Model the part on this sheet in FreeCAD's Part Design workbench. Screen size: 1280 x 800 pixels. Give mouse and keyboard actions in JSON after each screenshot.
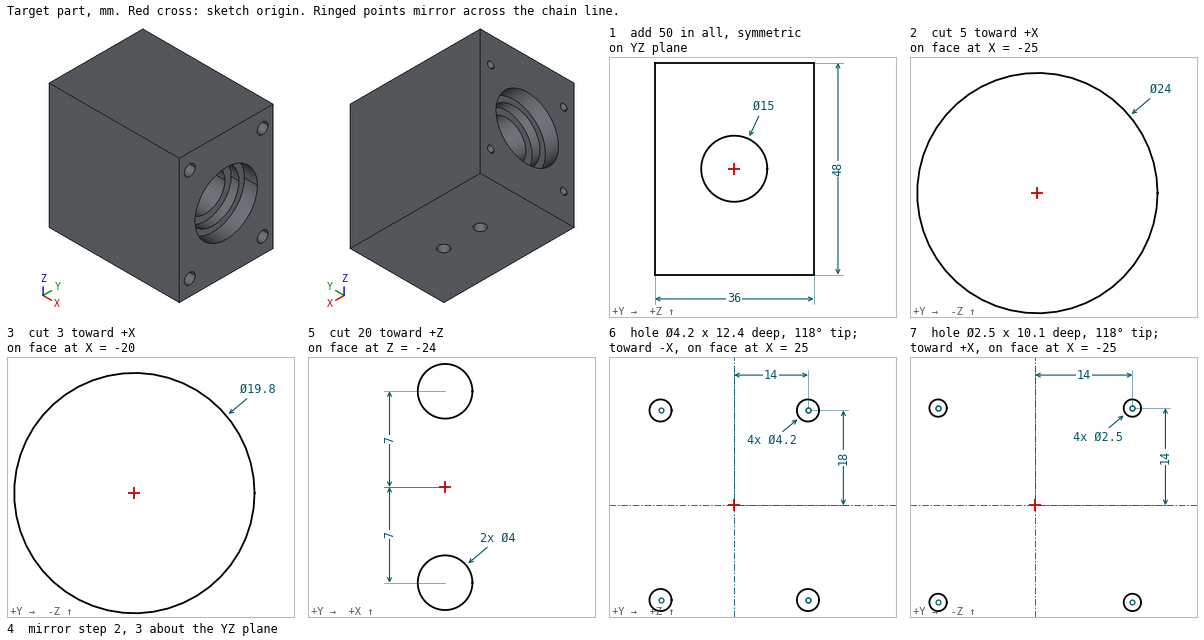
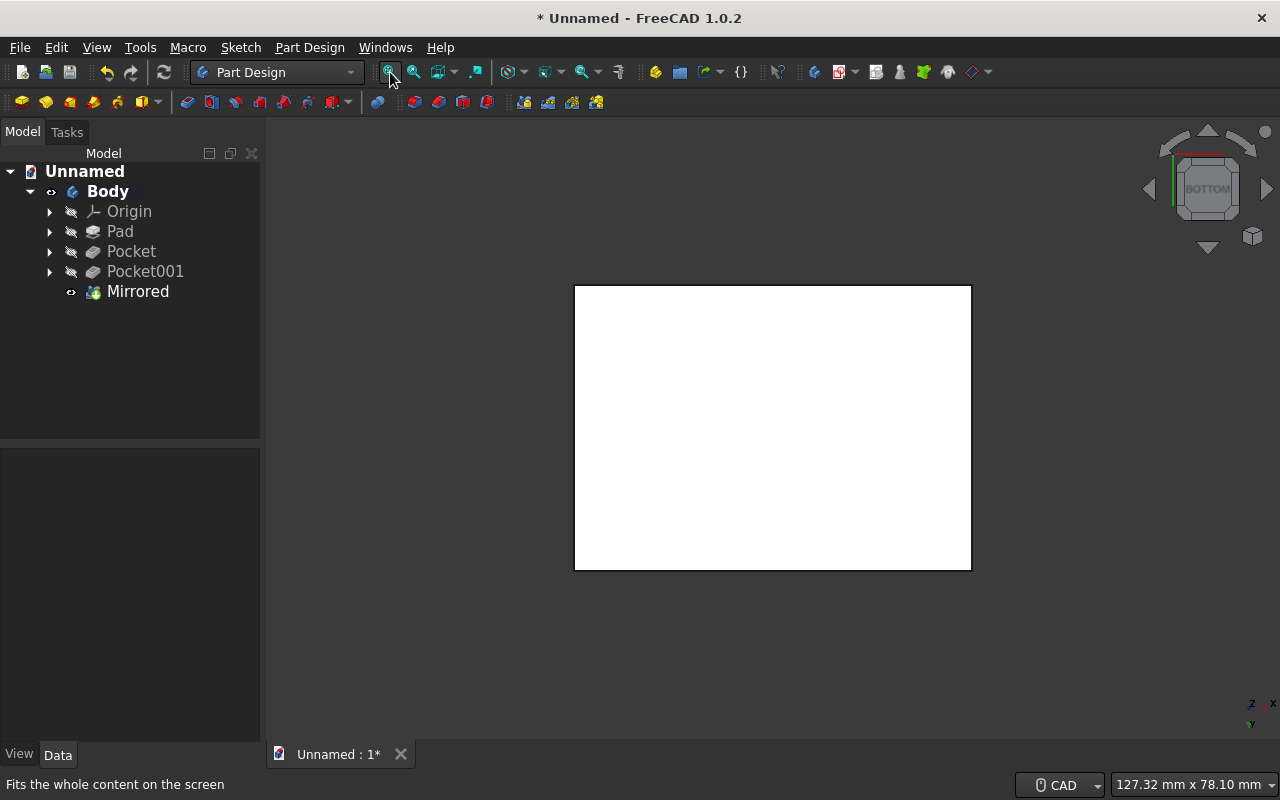
{"action": "left_click", "coordinate": [773, 427]}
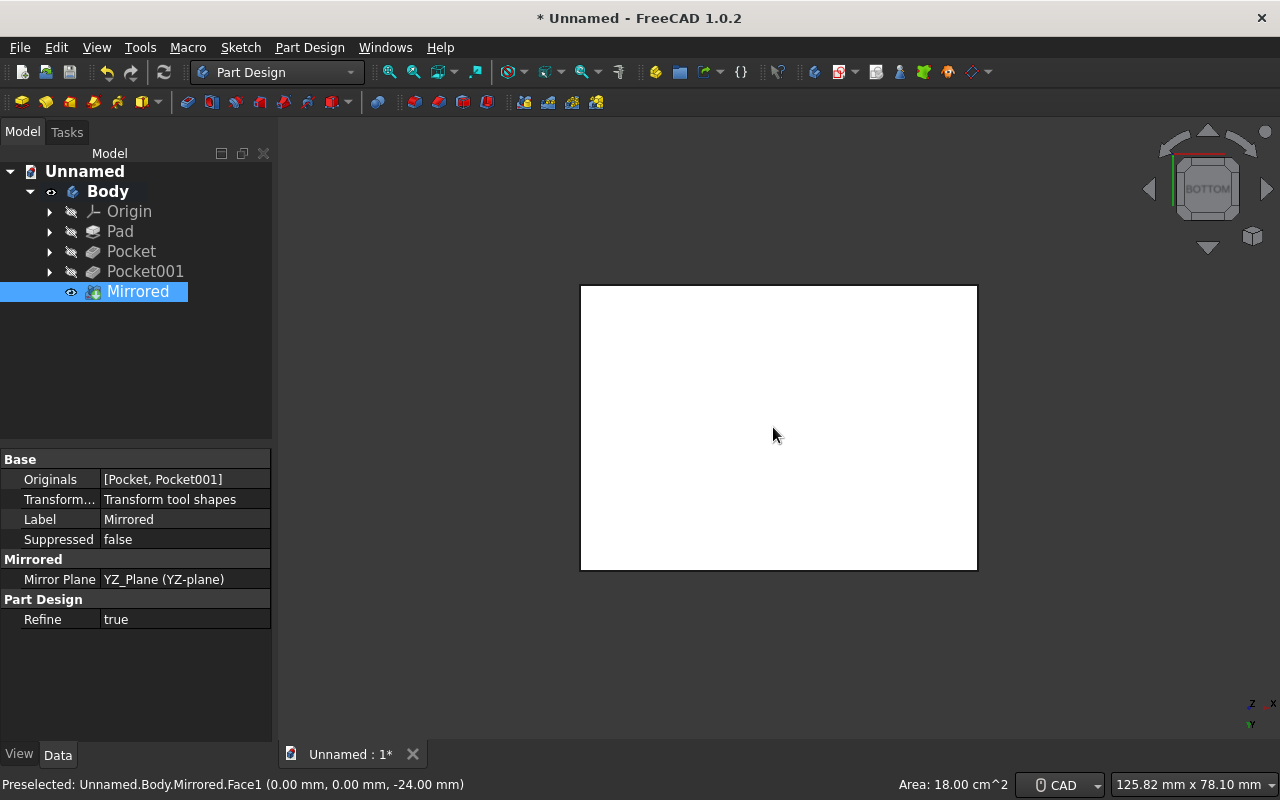
{"action": "left_click", "coordinate": [840, 72]}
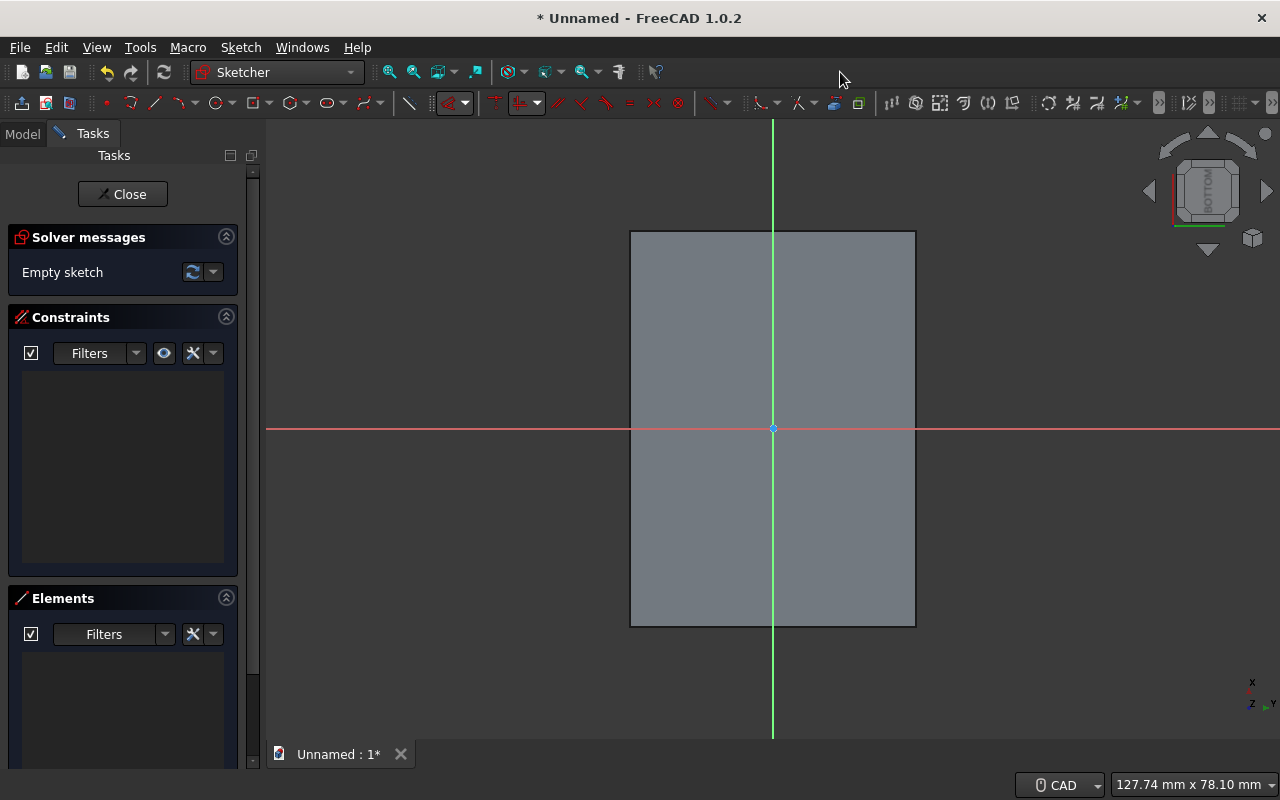
{"action": "scroll", "coordinate": [813, 429], "scroll_direction": "up", "scroll_amount": 5}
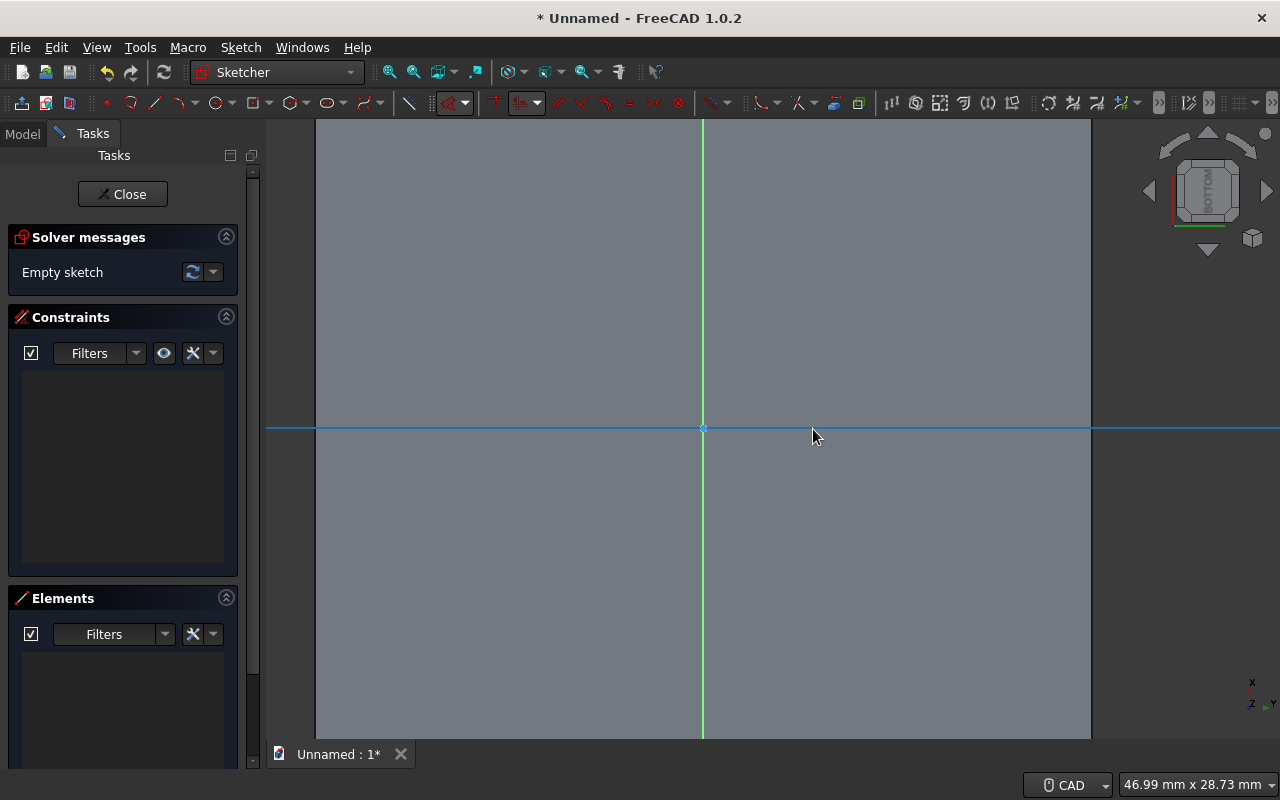
{"action": "left_click", "coordinate": [216, 104]}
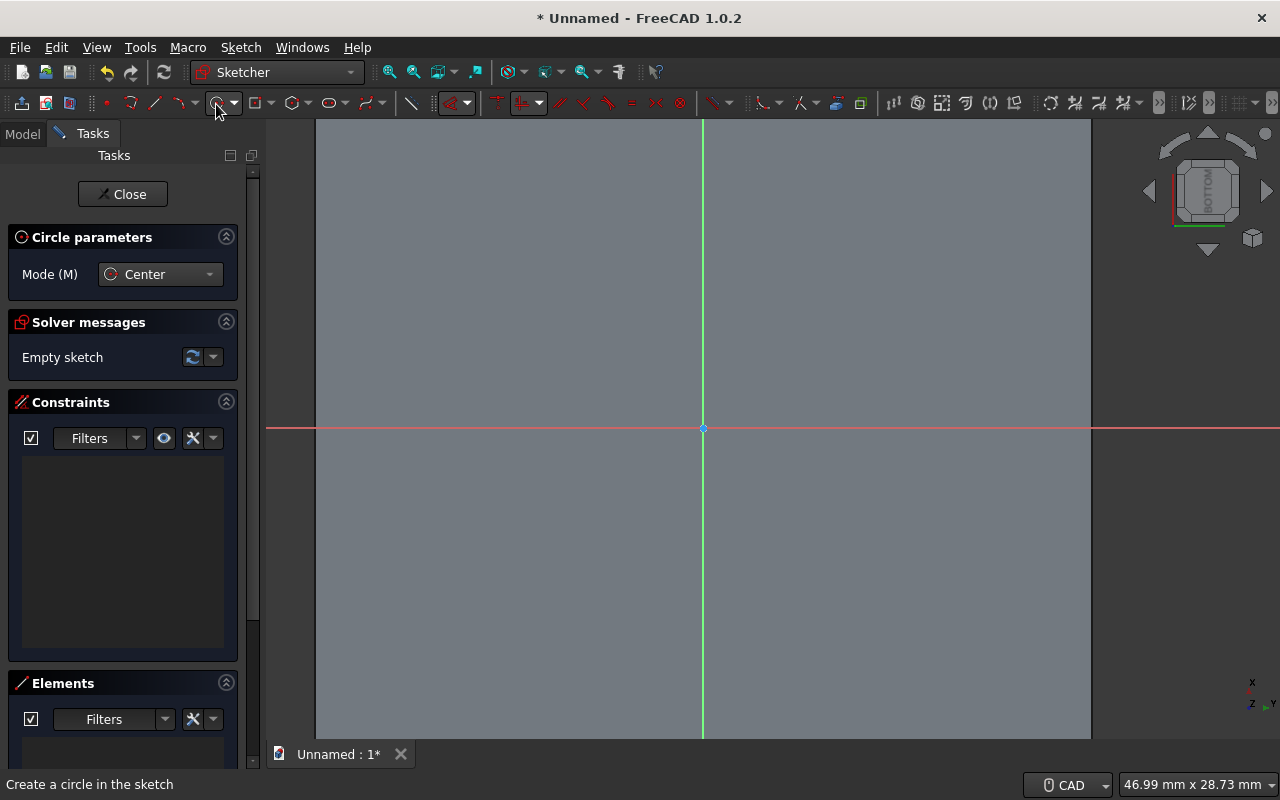
{"action": "left_click", "coordinate": [703, 579]}
{"action": "left_click", "coordinate": [734, 549]}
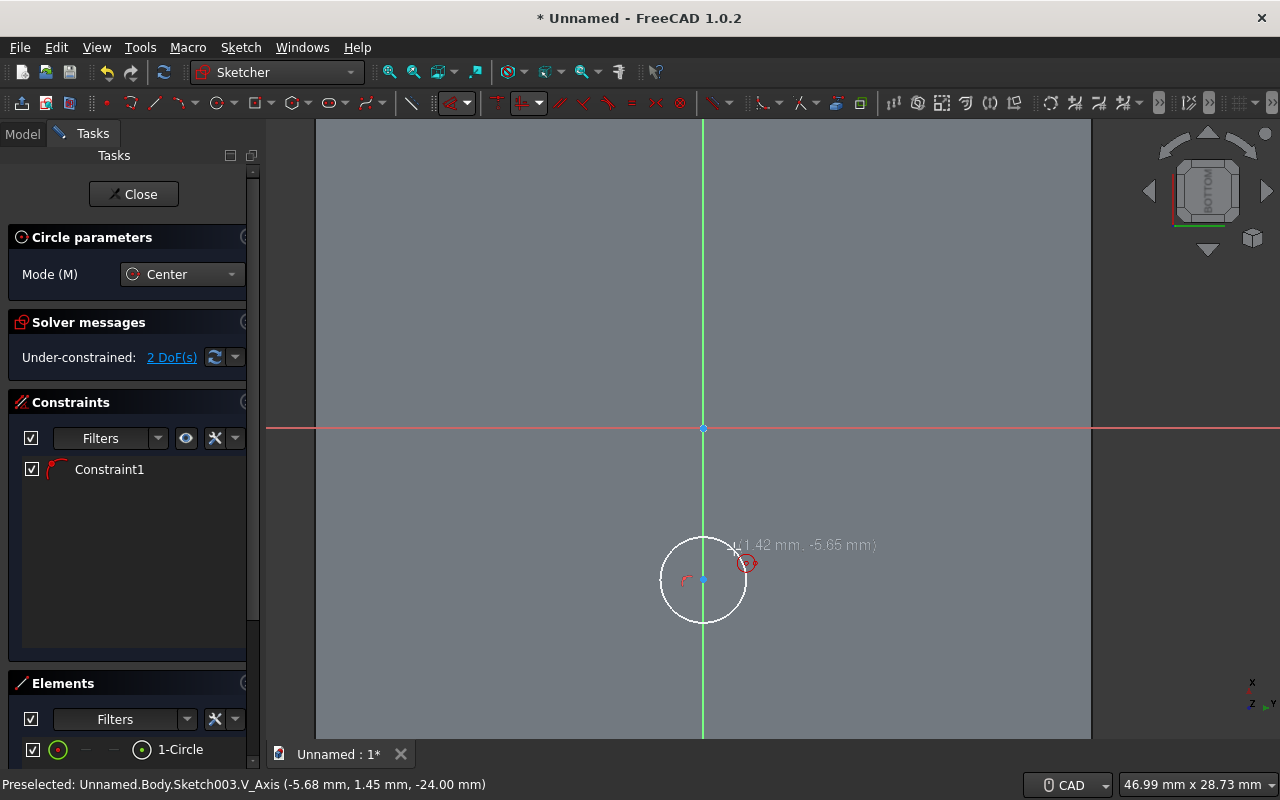
{"action": "left_click", "coordinate": [703, 277]}
{"action": "left_click", "coordinate": [734, 247]}
{"action": "key", "text": "Escape"}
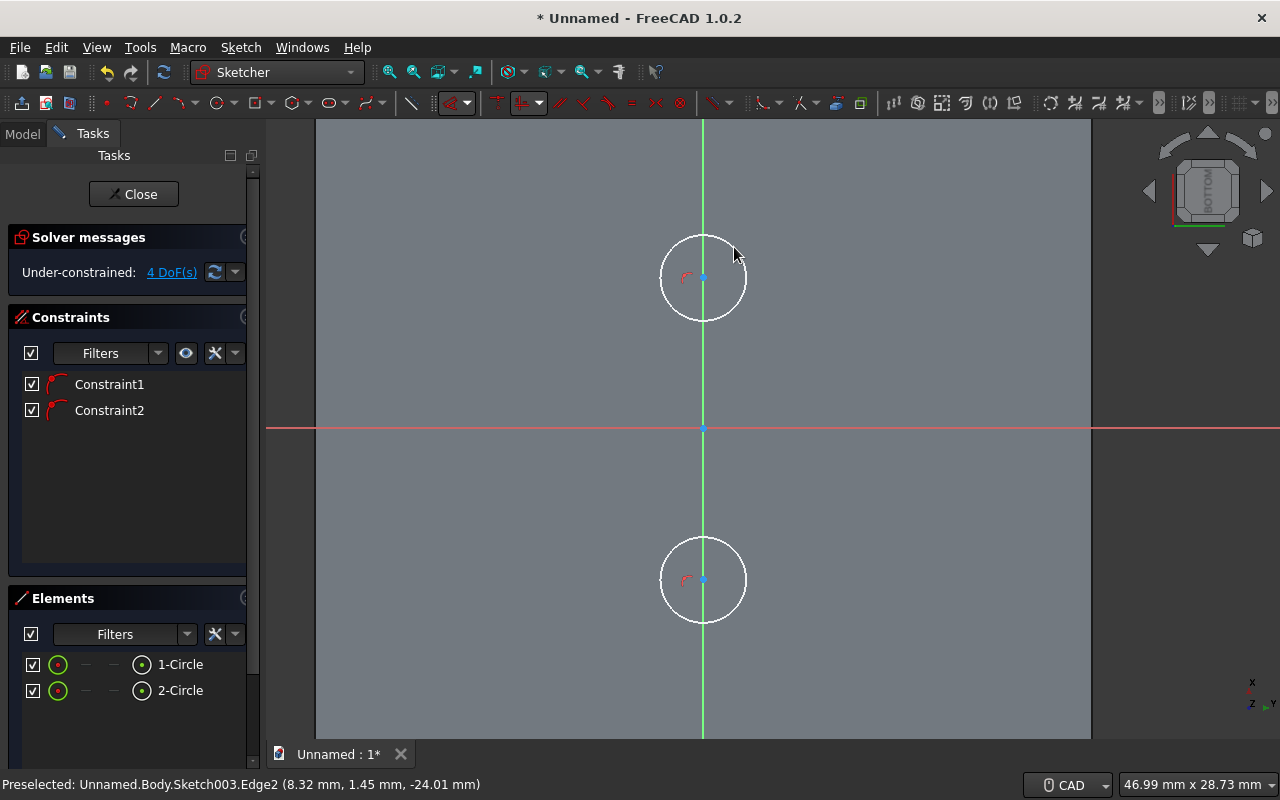
{"action": "left_click", "coordinate": [734, 550]}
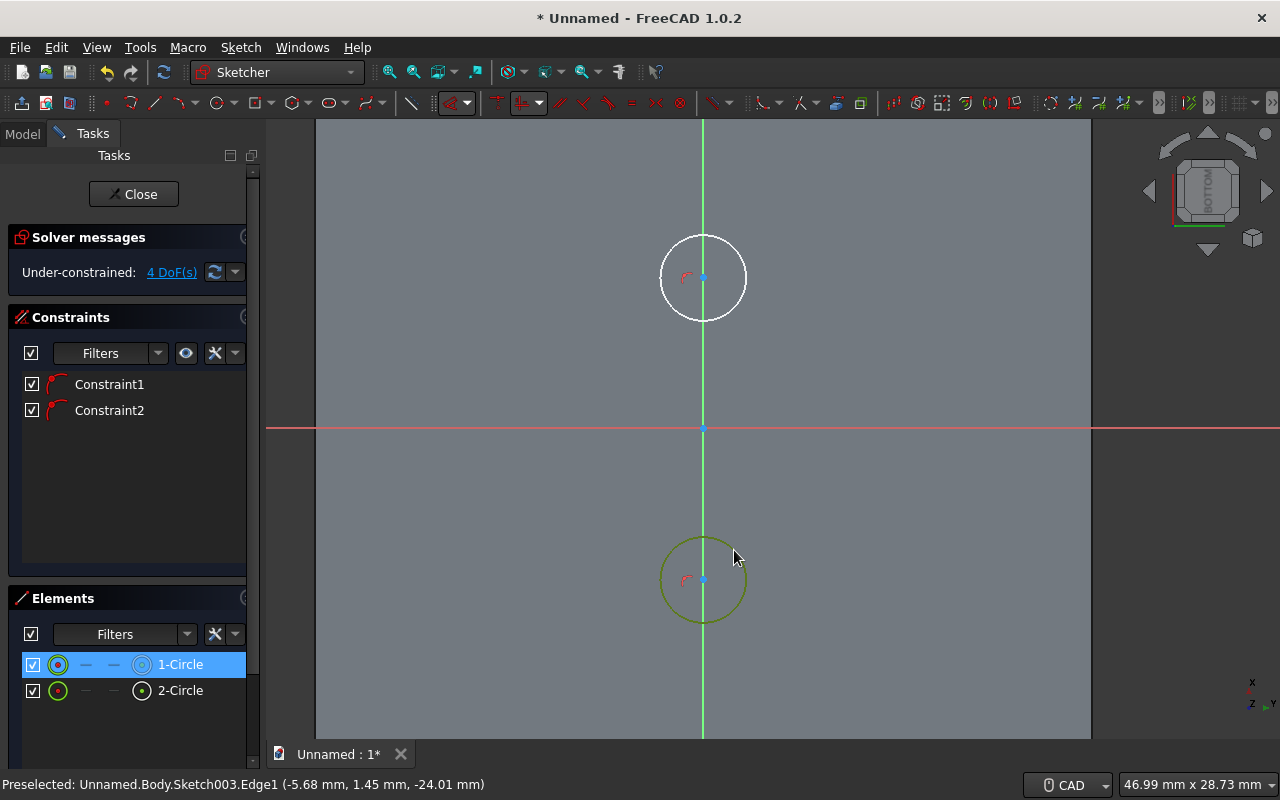
{"action": "left_click", "coordinate": [734, 248]}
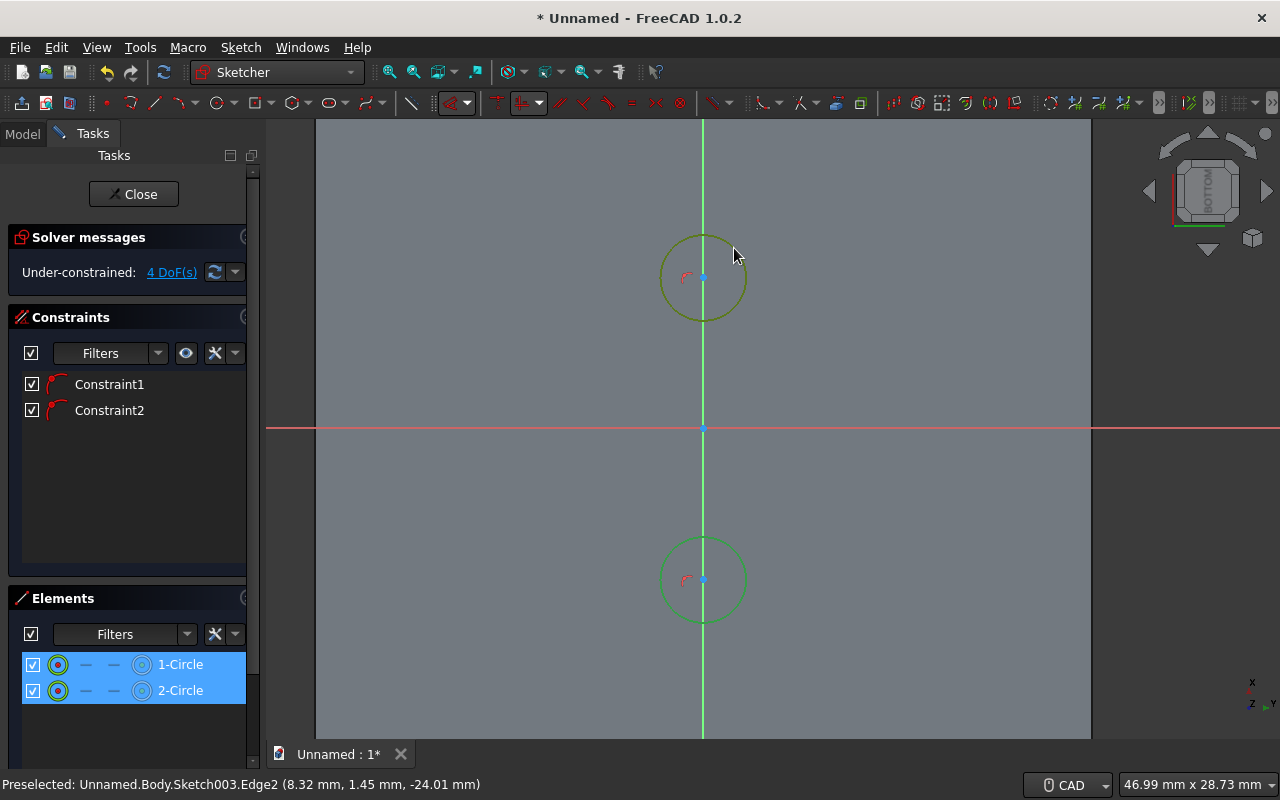
{"action": "left_click", "coordinate": [632, 104]}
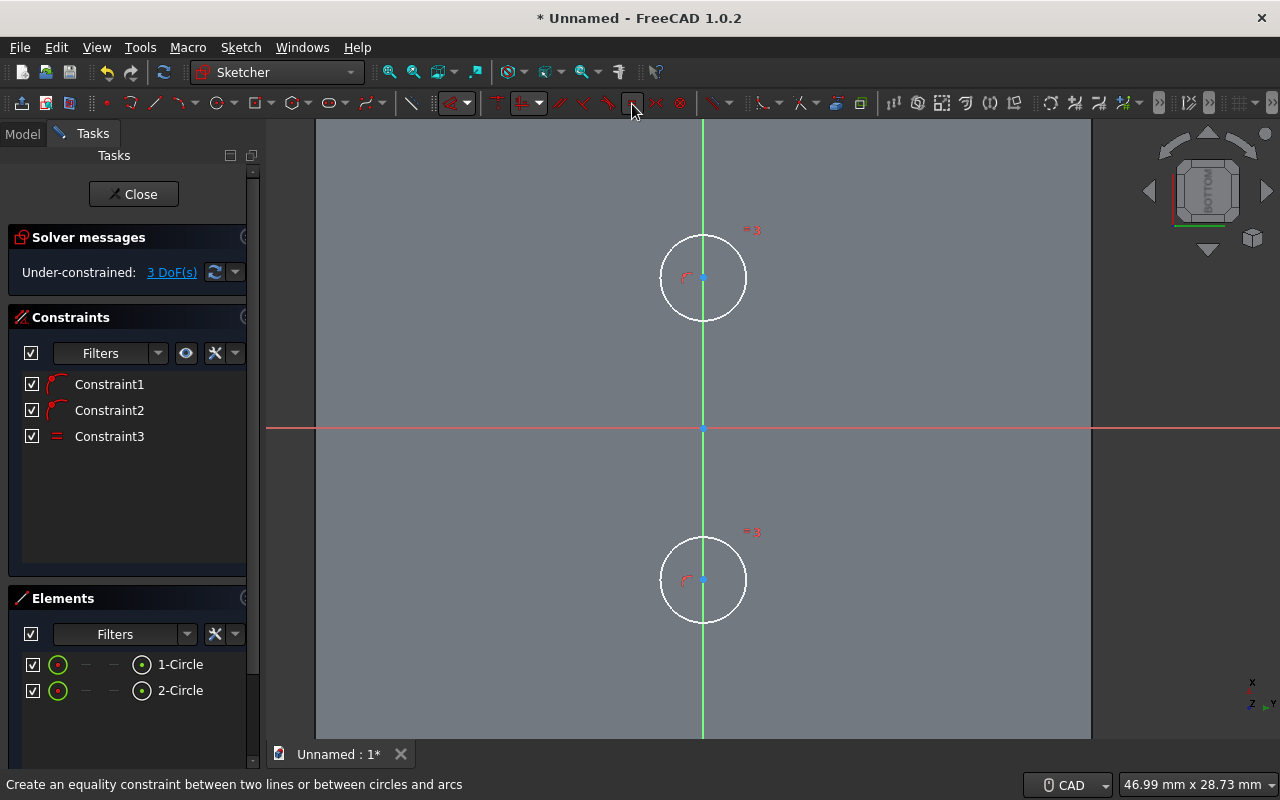
{"action": "left_click", "coordinate": [734, 550]}